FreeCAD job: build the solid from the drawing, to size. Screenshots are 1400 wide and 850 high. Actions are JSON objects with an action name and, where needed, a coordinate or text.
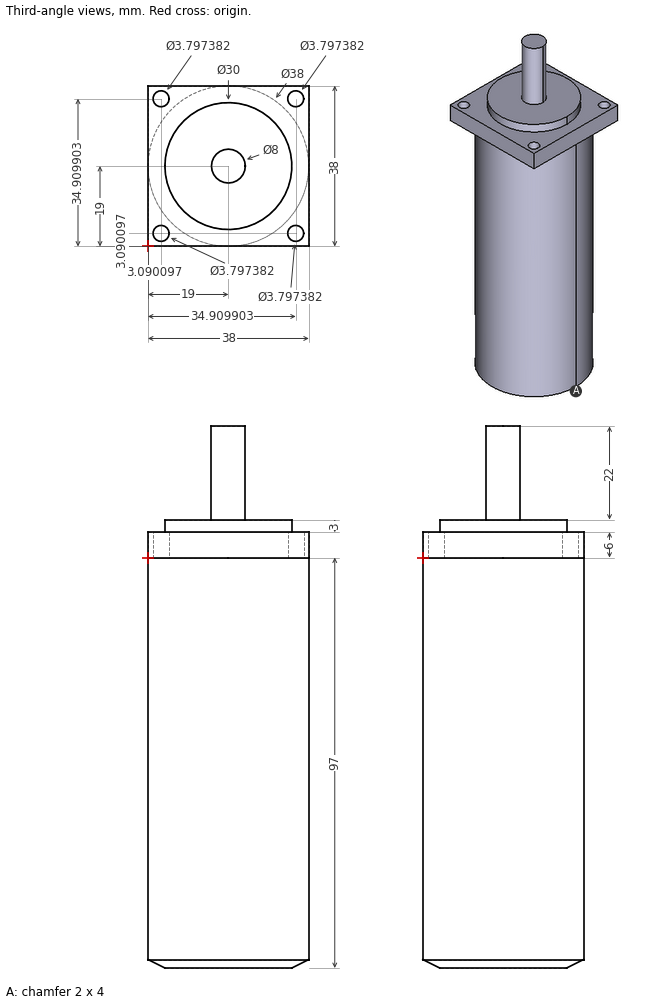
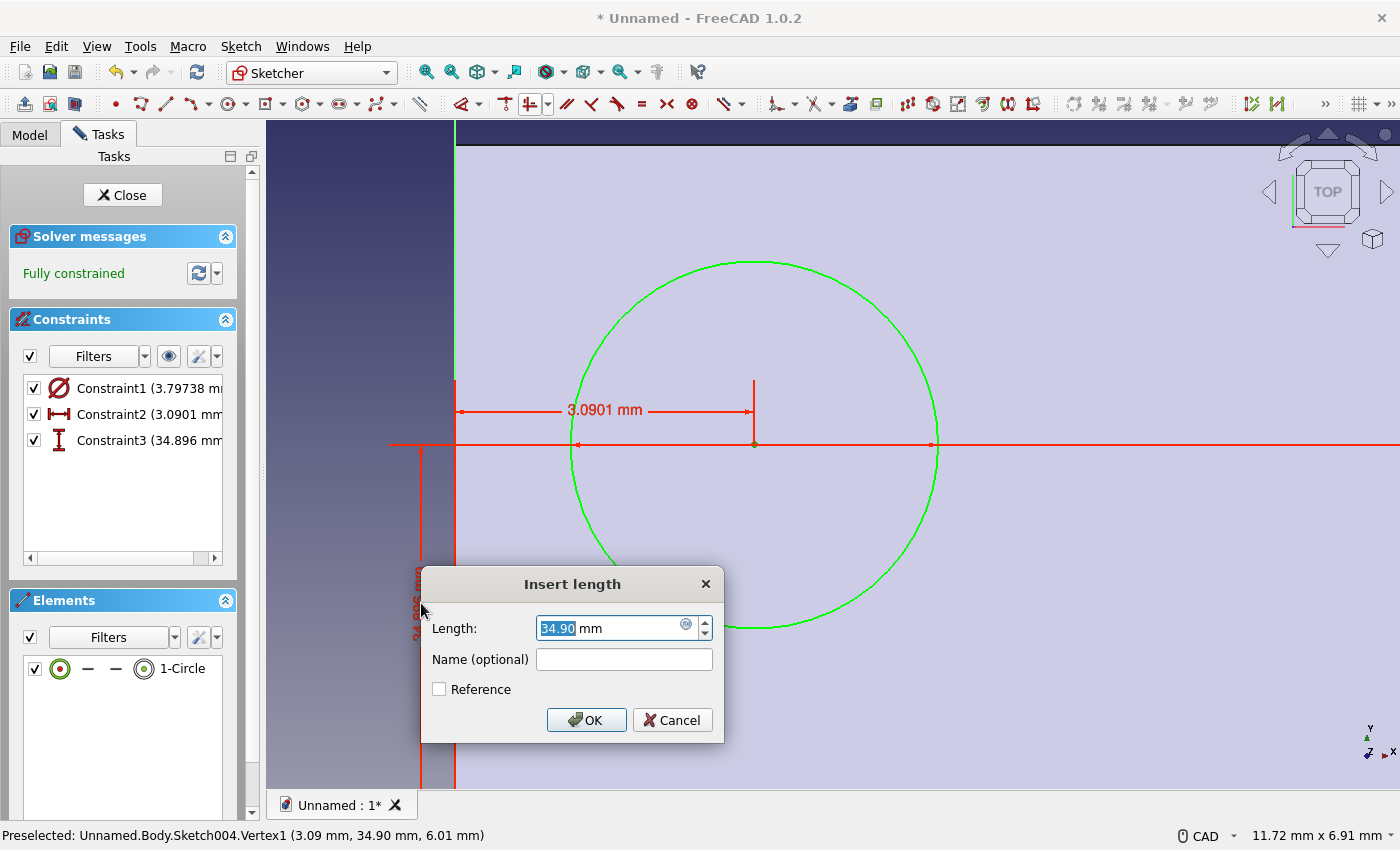
{"action": "type", "text": "34.909903"}
{"action": "key", "text": "Return"}
{"action": "key", "text": "Escape"}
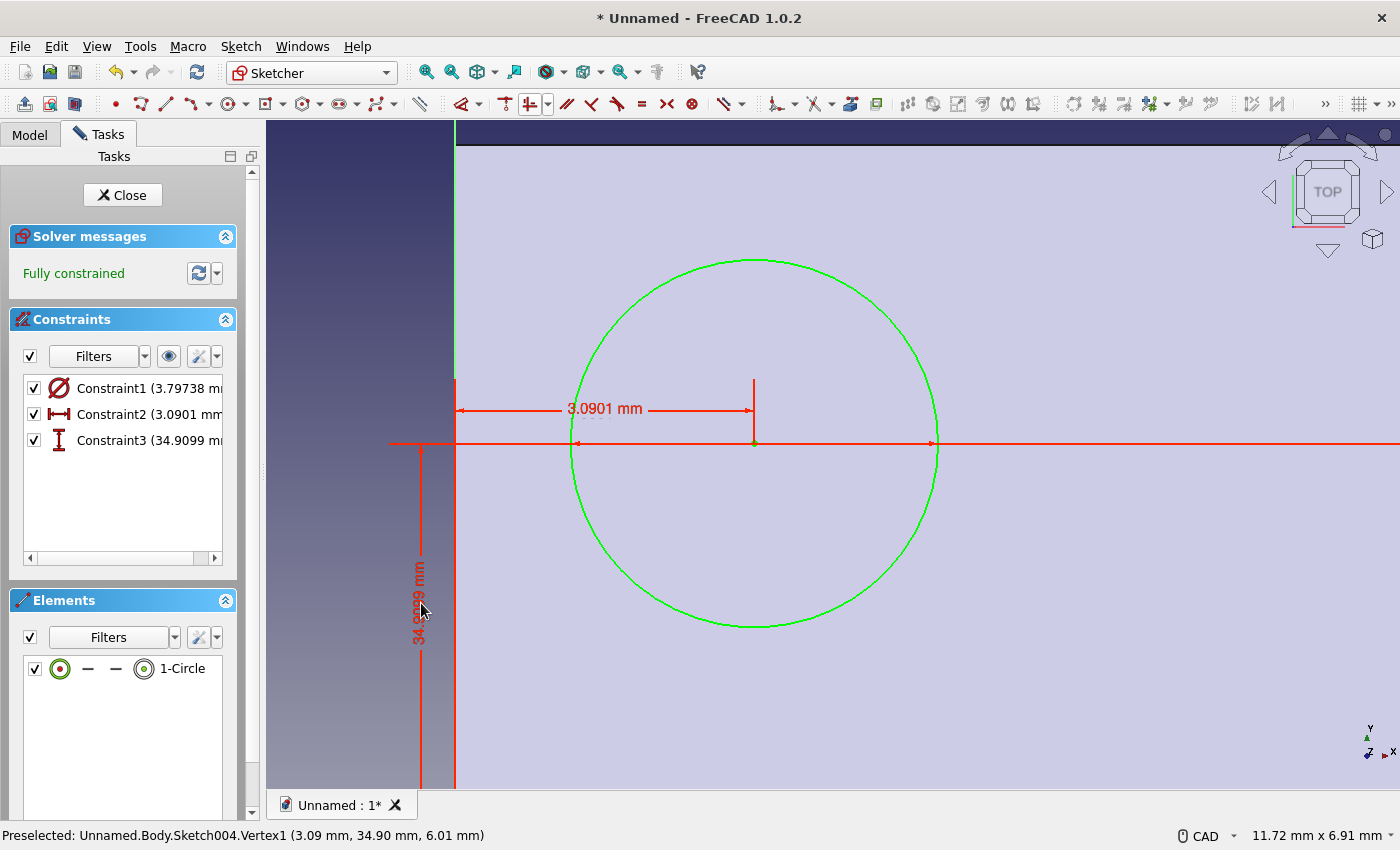
{"action": "left_click", "coordinate": [123, 195]}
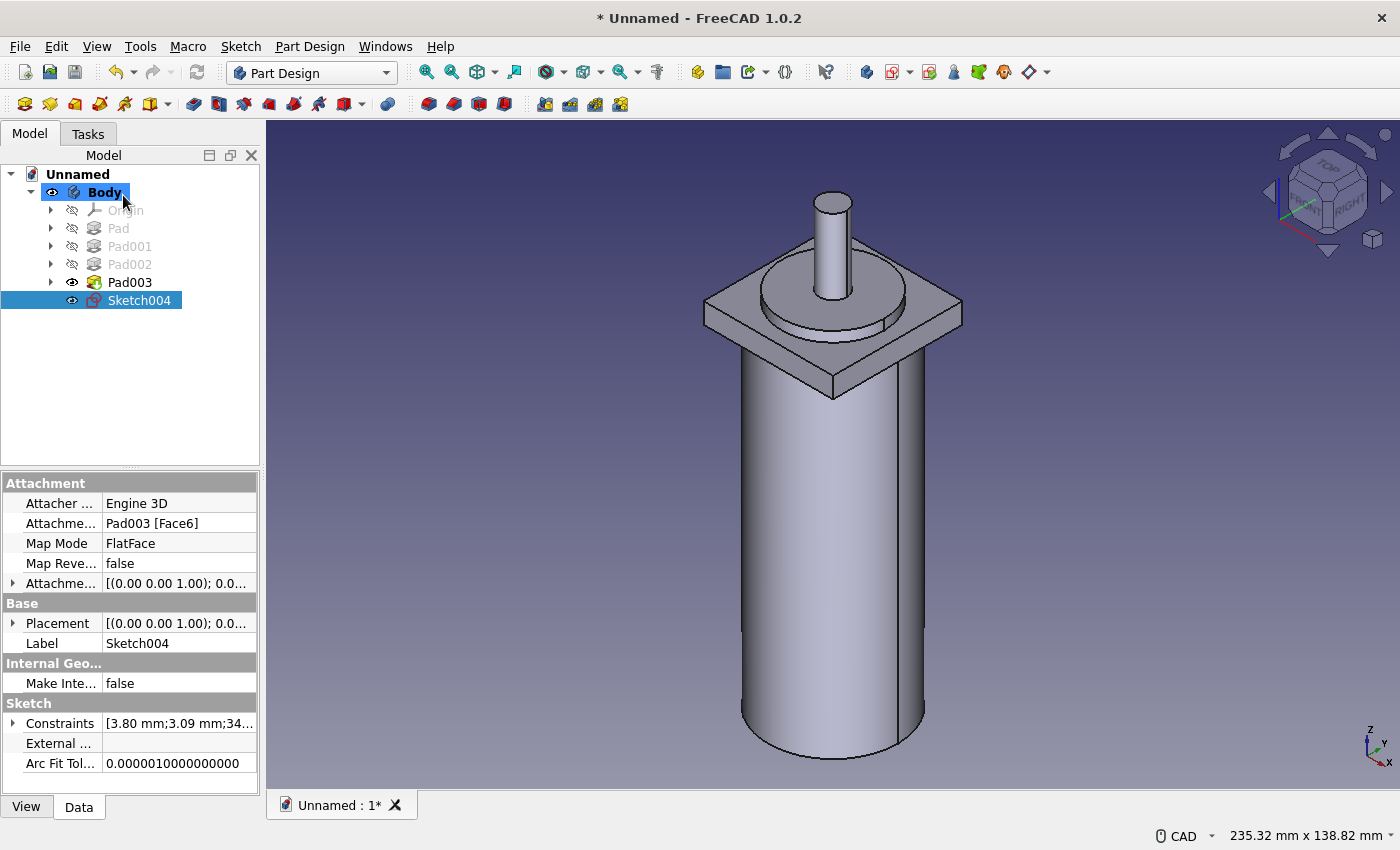
{"action": "left_click", "coordinate": [194, 104]}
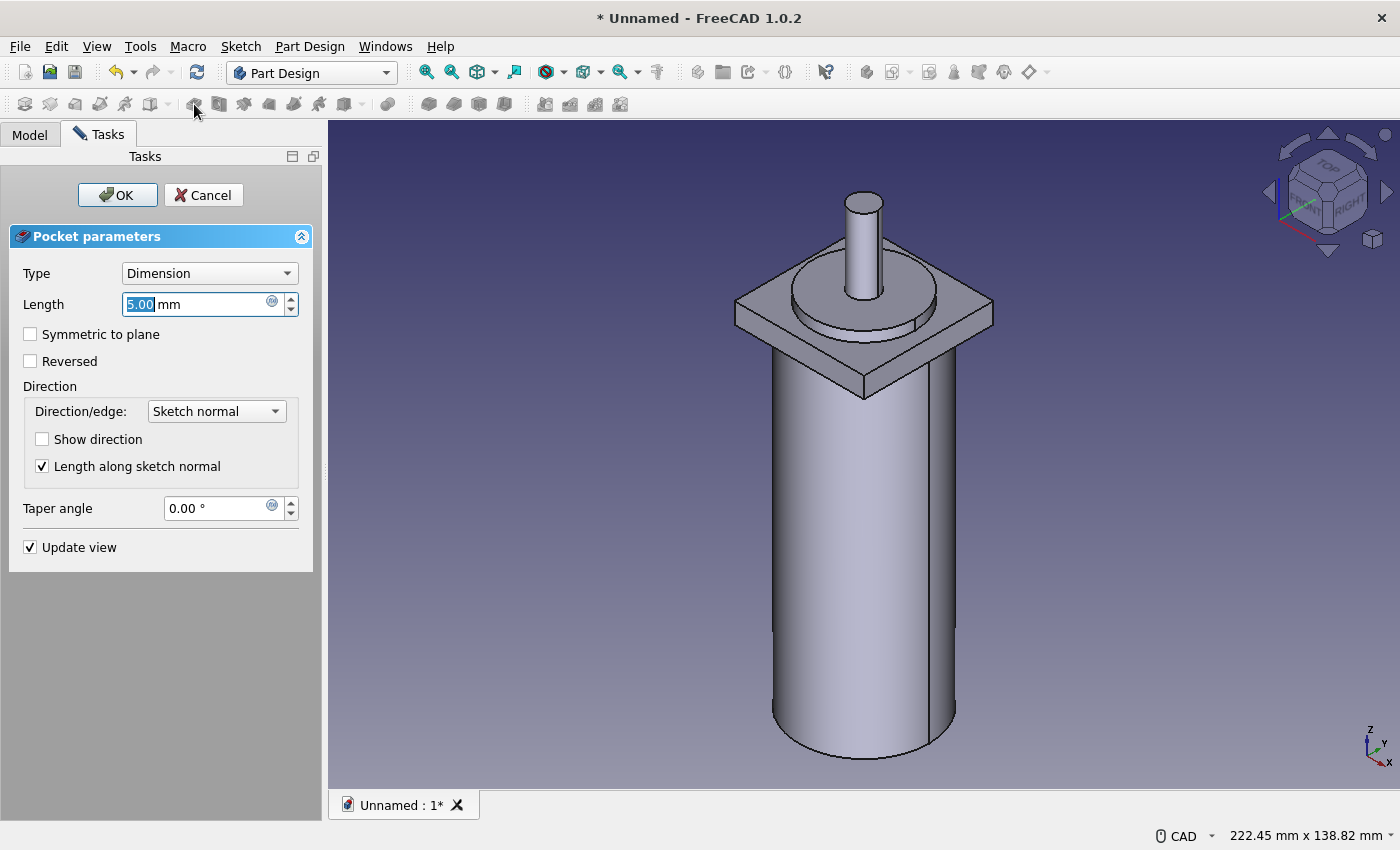
{"action": "left_click", "coordinate": [210, 274]}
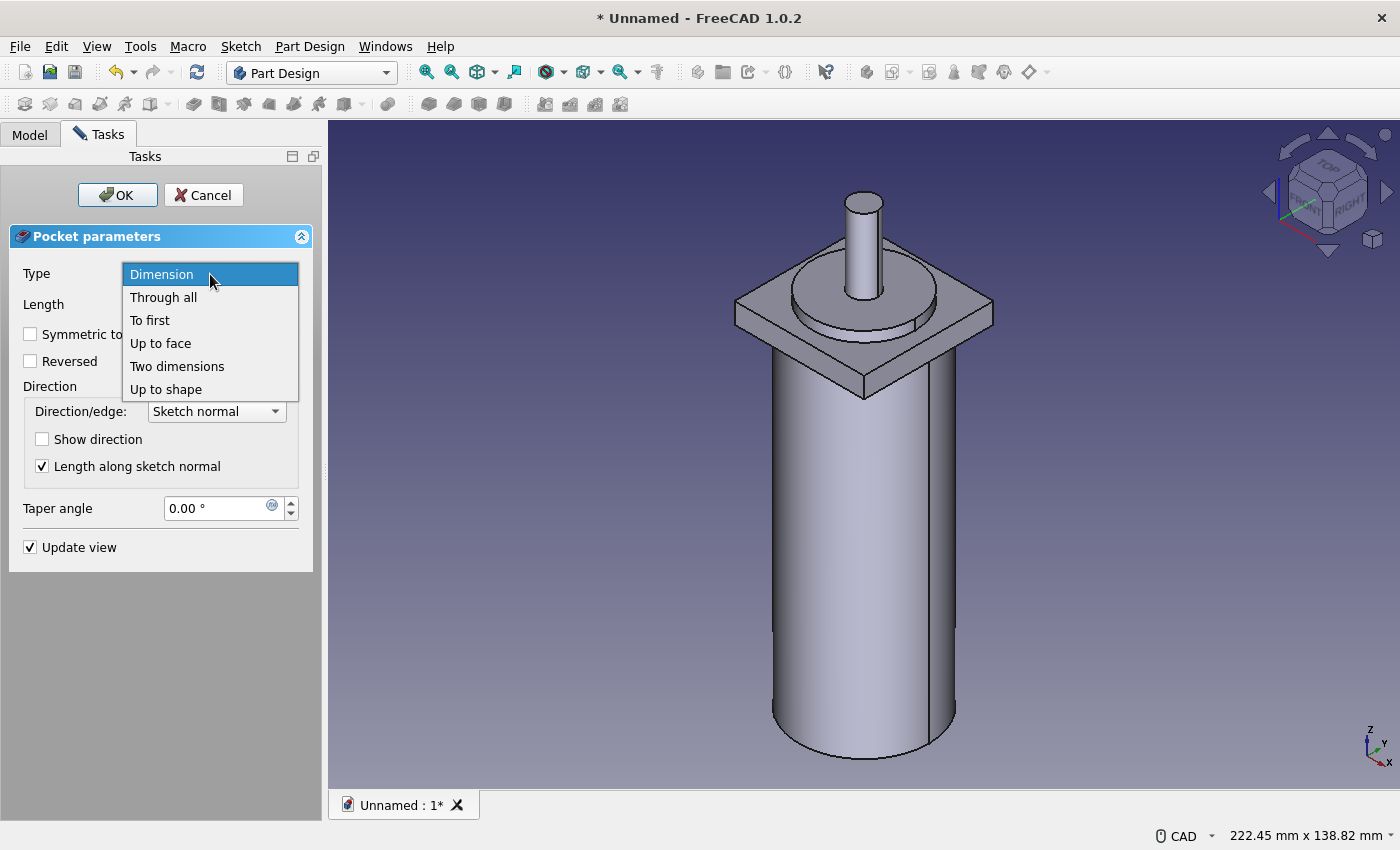
{"action": "left_click", "coordinate": [208, 320]}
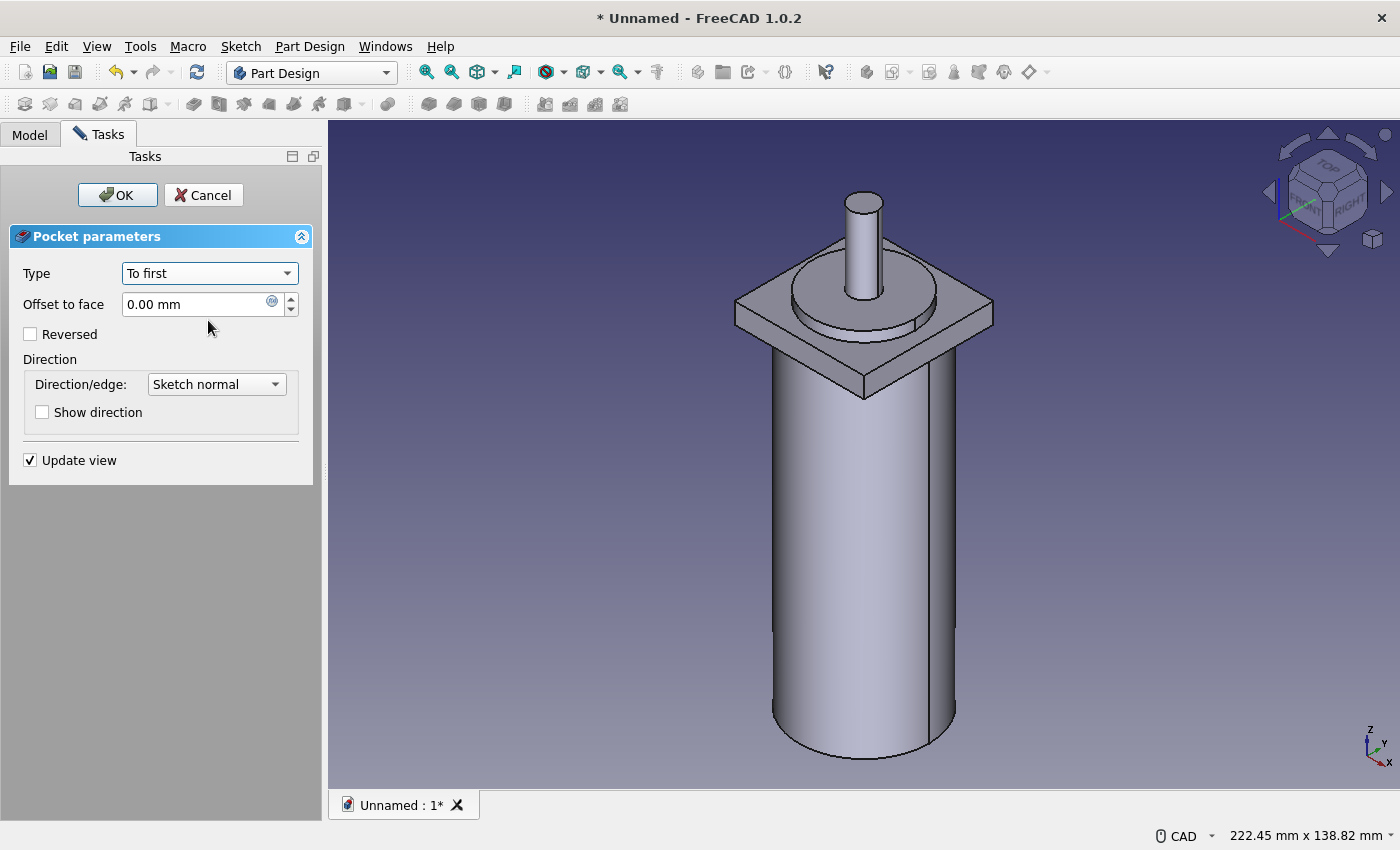
{"action": "left_click", "coordinate": [118, 195]}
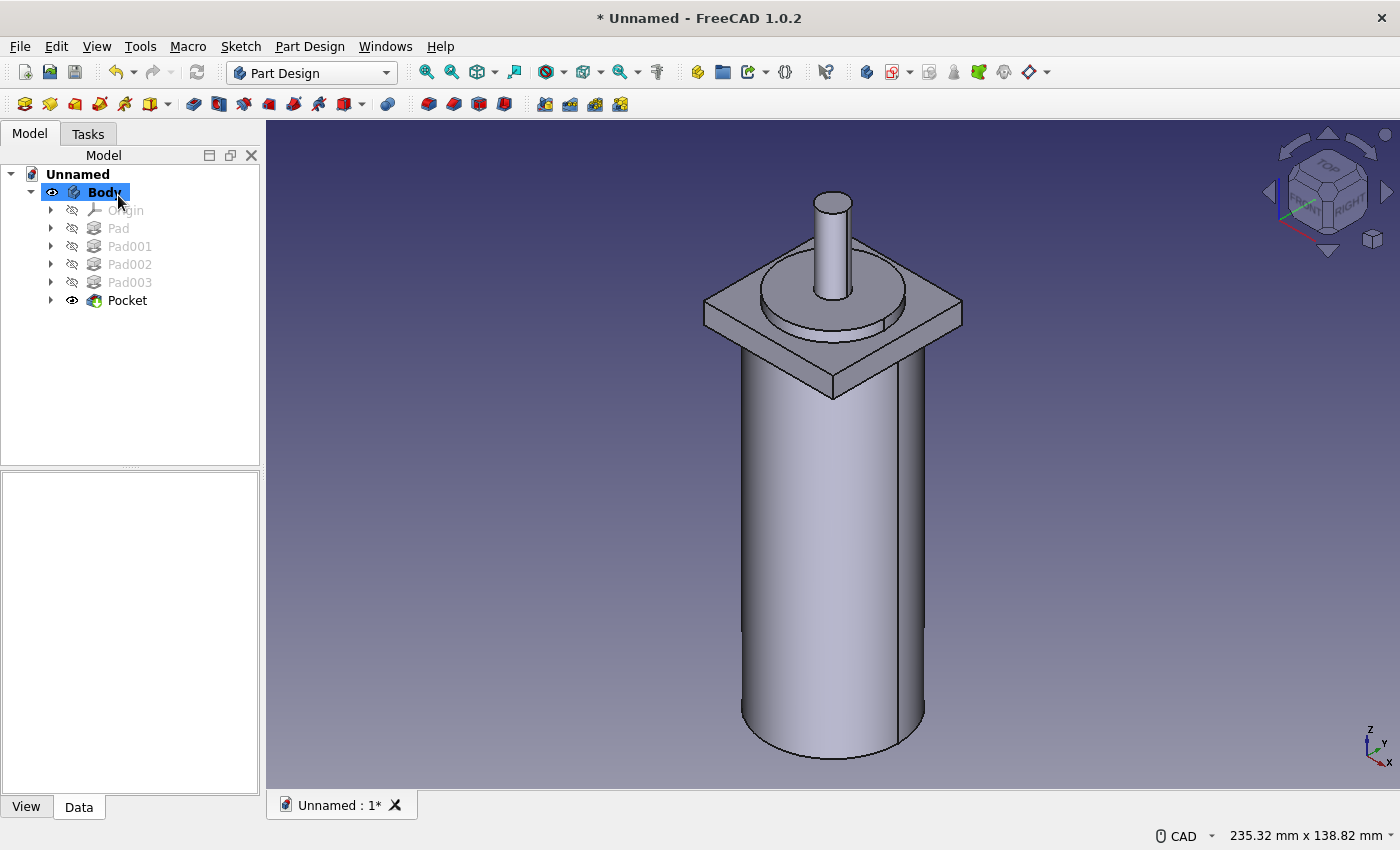
{"action": "left_click", "coordinate": [944, 300]}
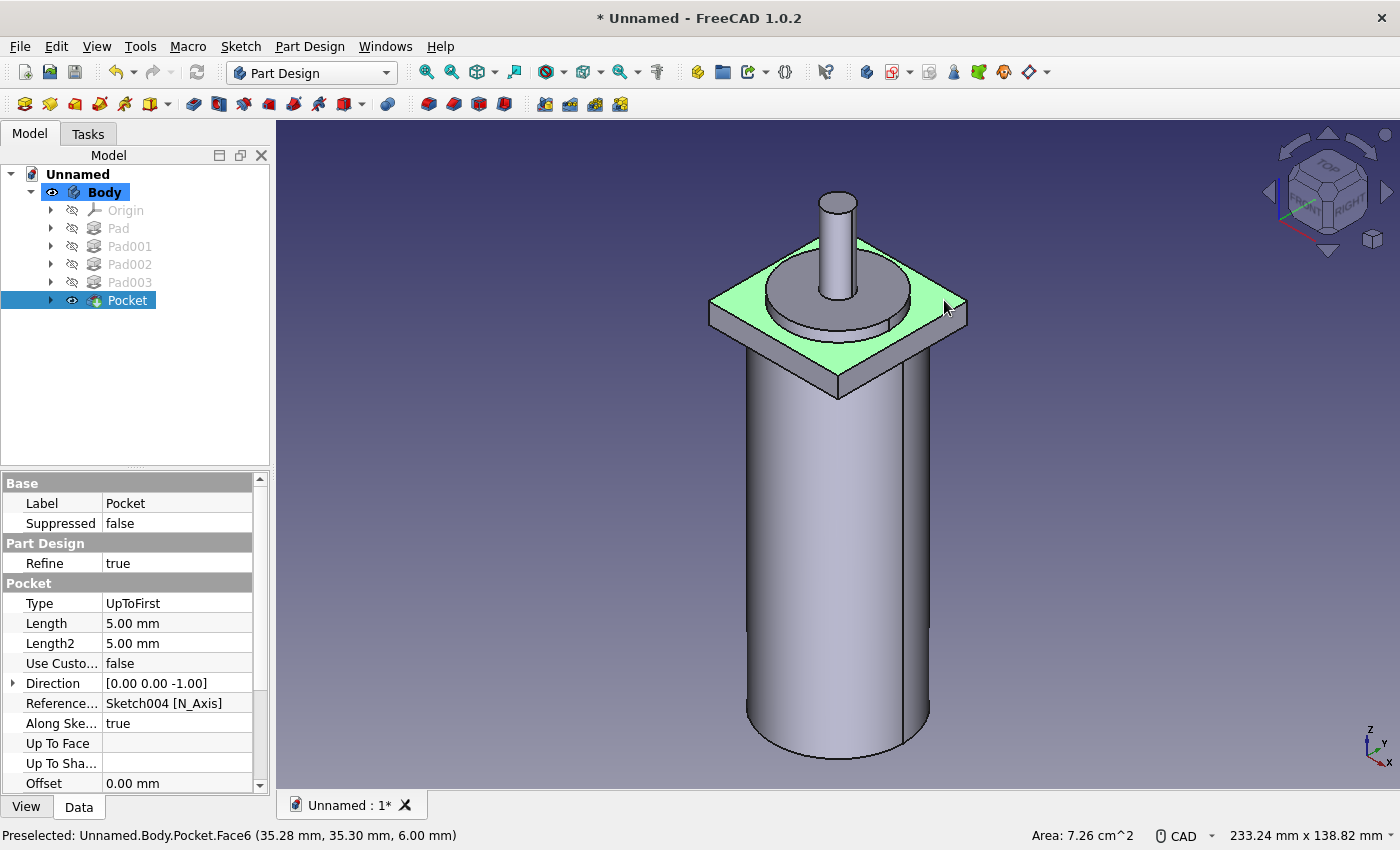
{"action": "left_click", "coordinate": [892, 72]}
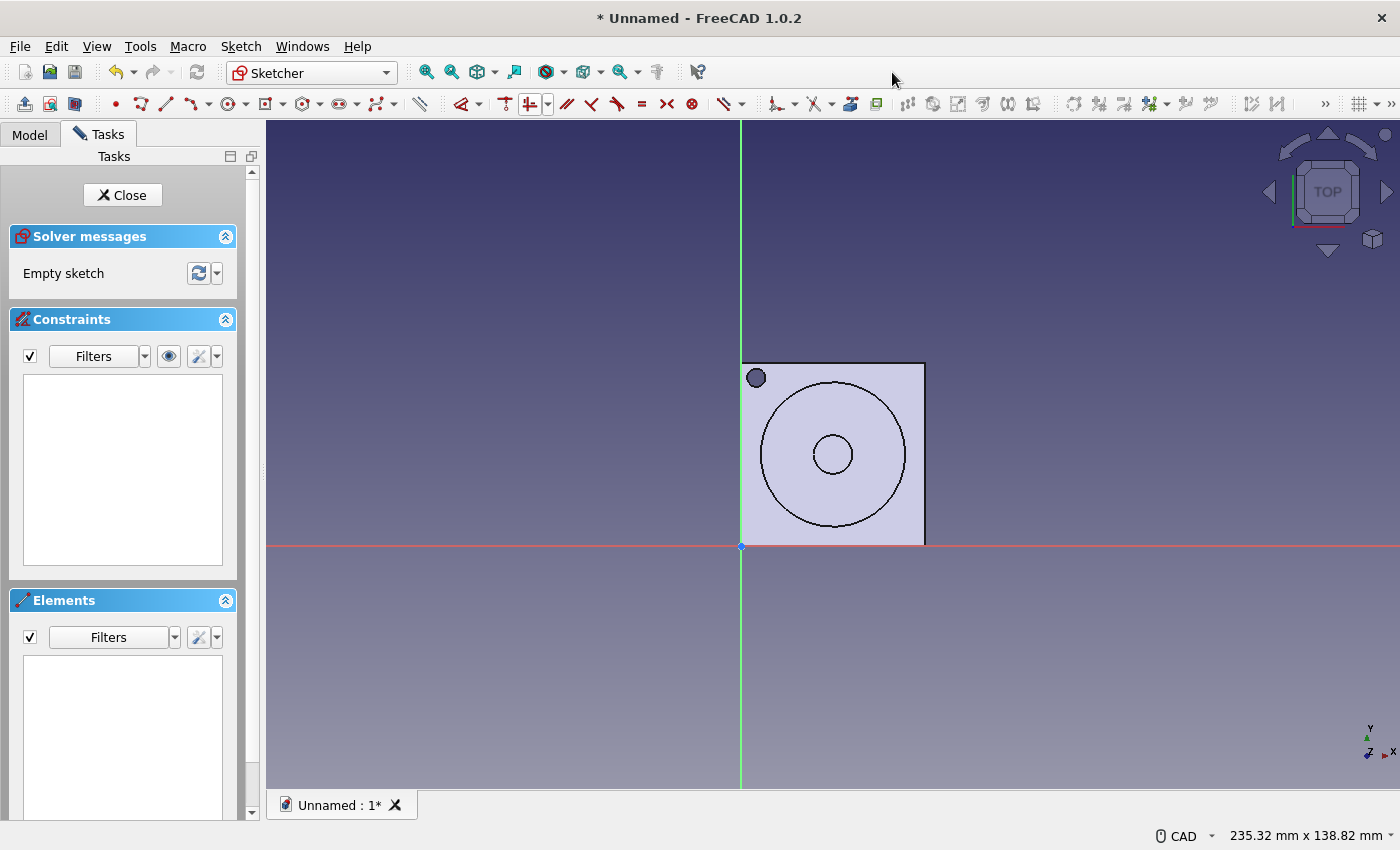
{"action": "key", "text": "q s"}